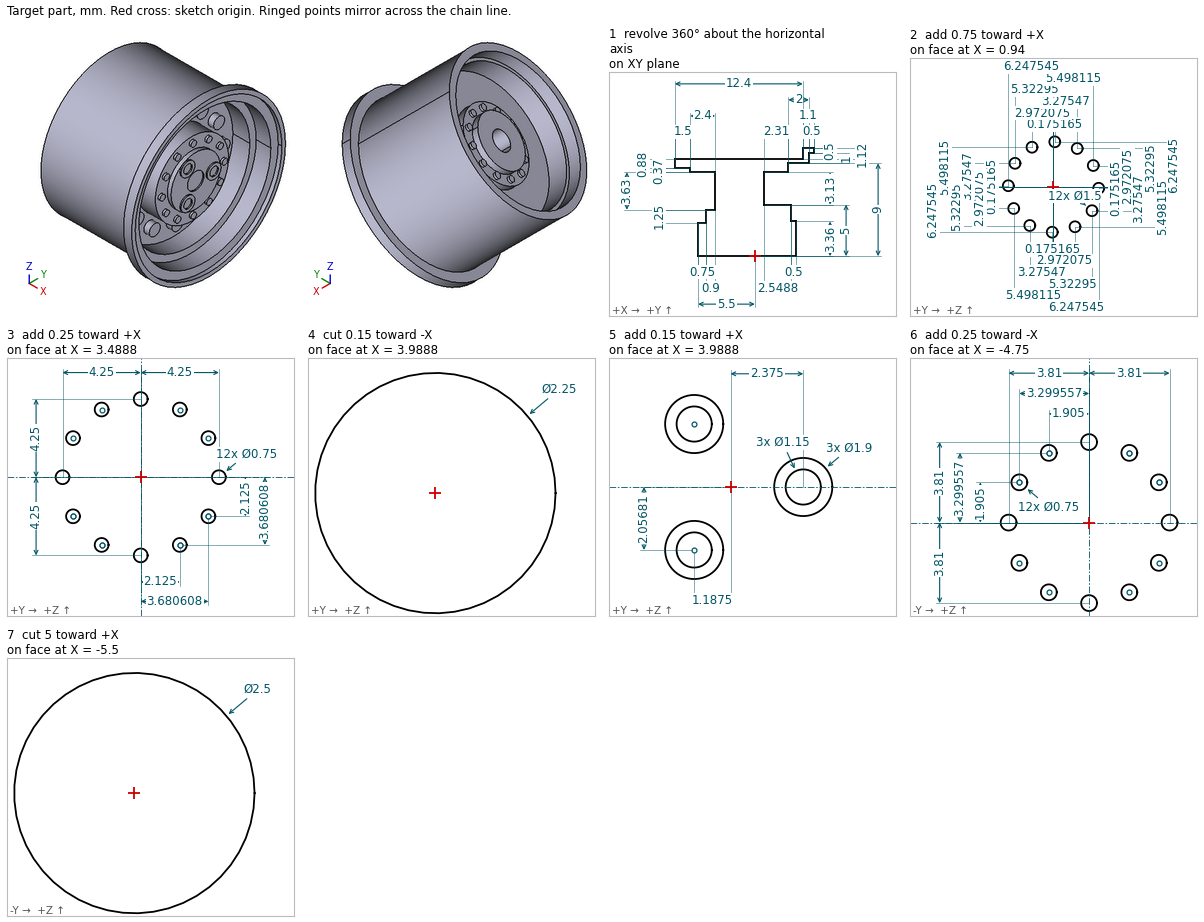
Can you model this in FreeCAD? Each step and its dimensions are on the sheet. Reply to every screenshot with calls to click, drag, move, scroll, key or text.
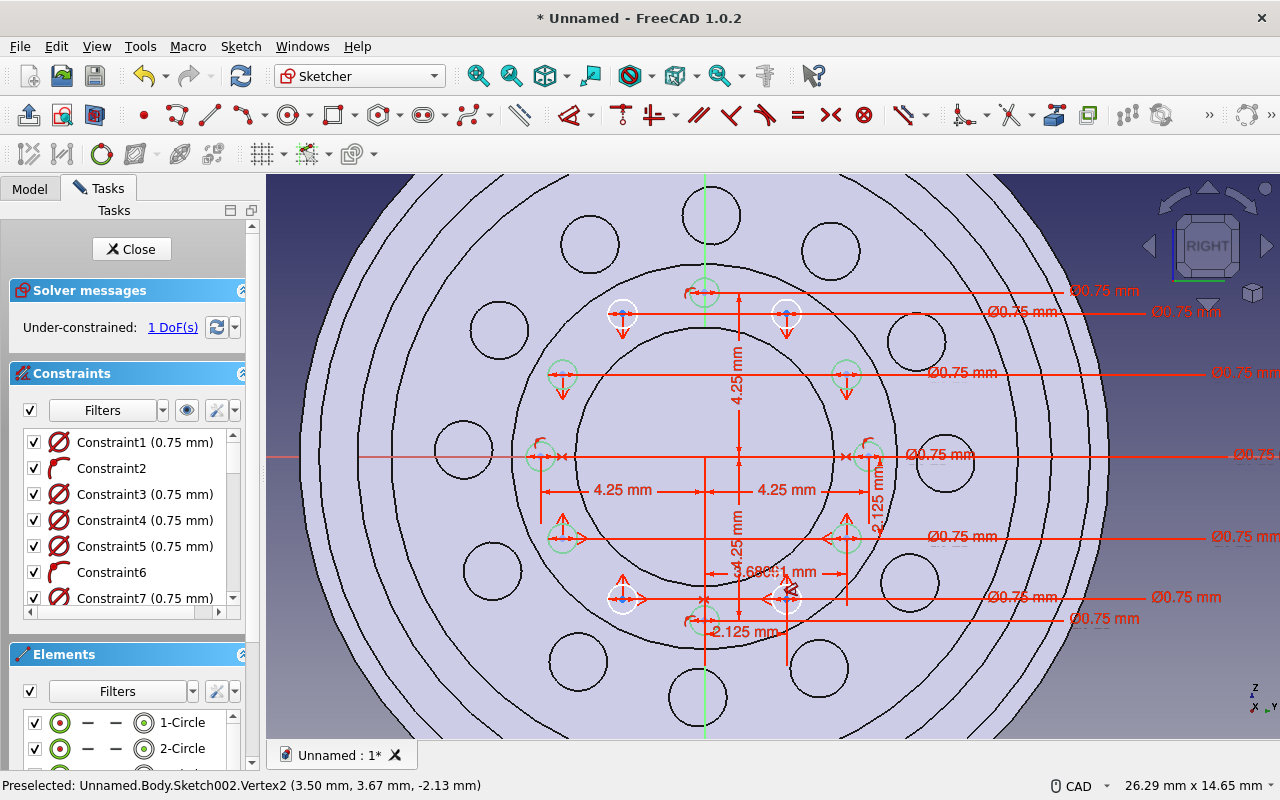
click(787, 599)
click(821, 528)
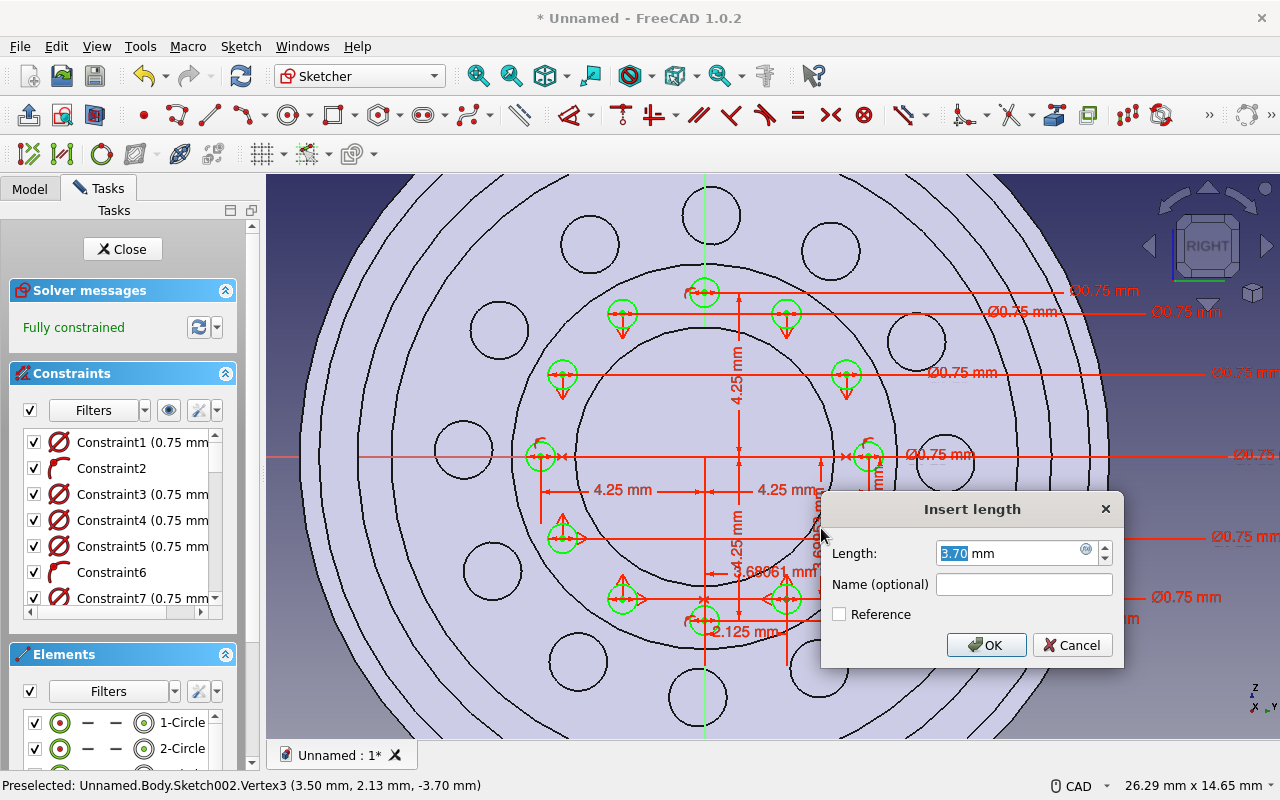
text(3.680608)
key(Return)
key(Escape)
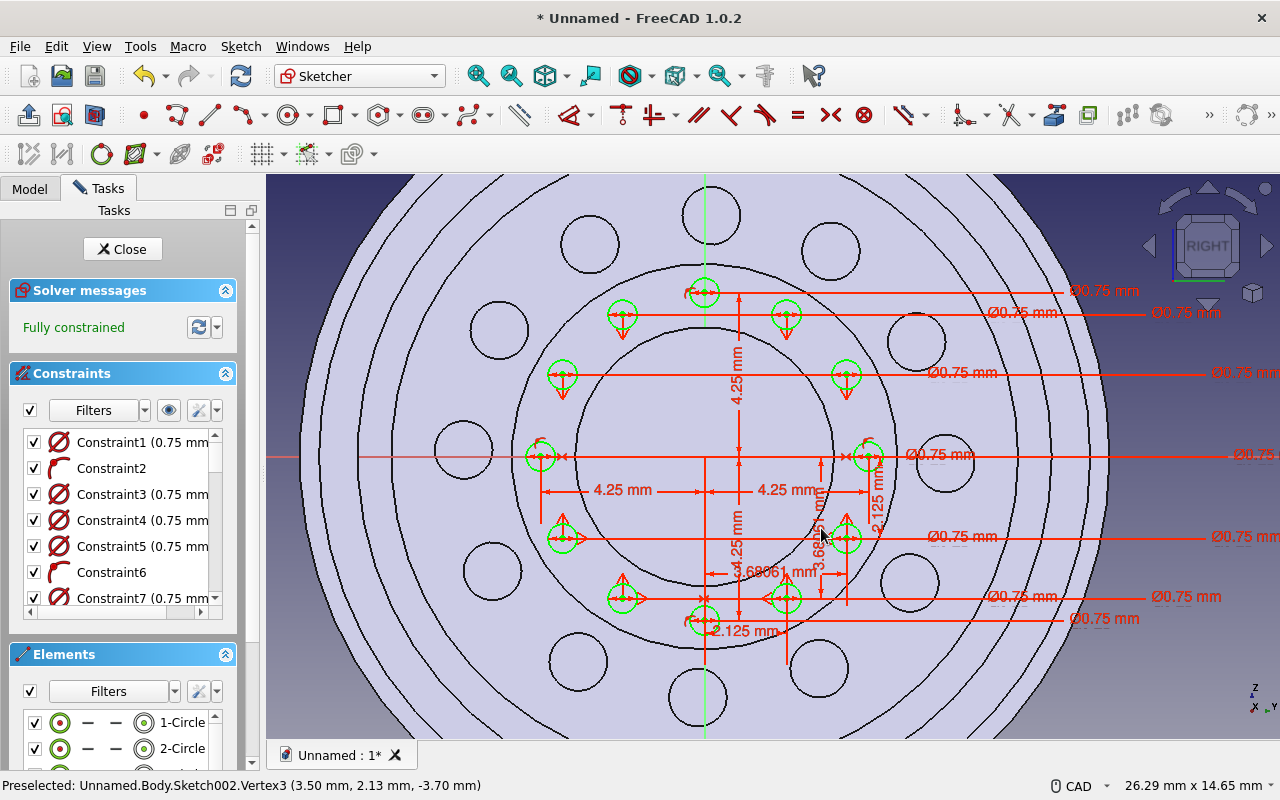
click(123, 249)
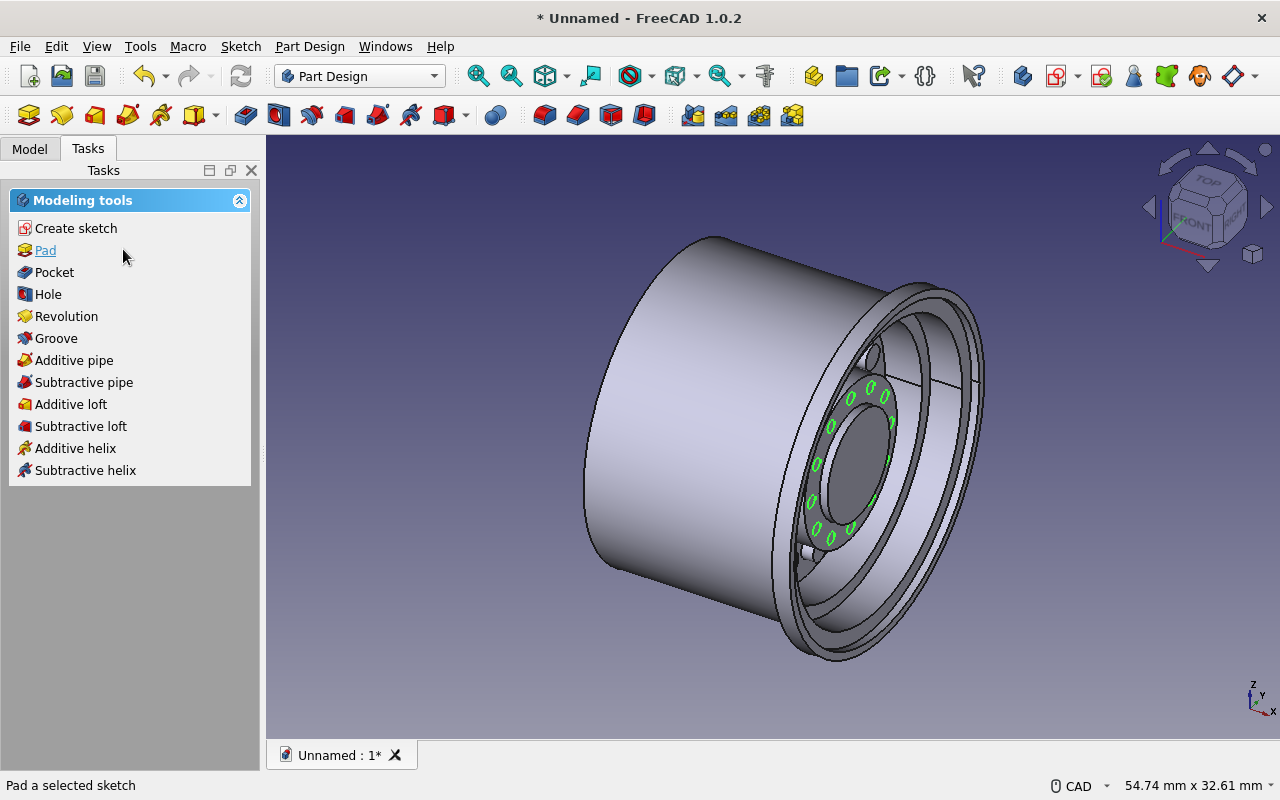
click(29, 116)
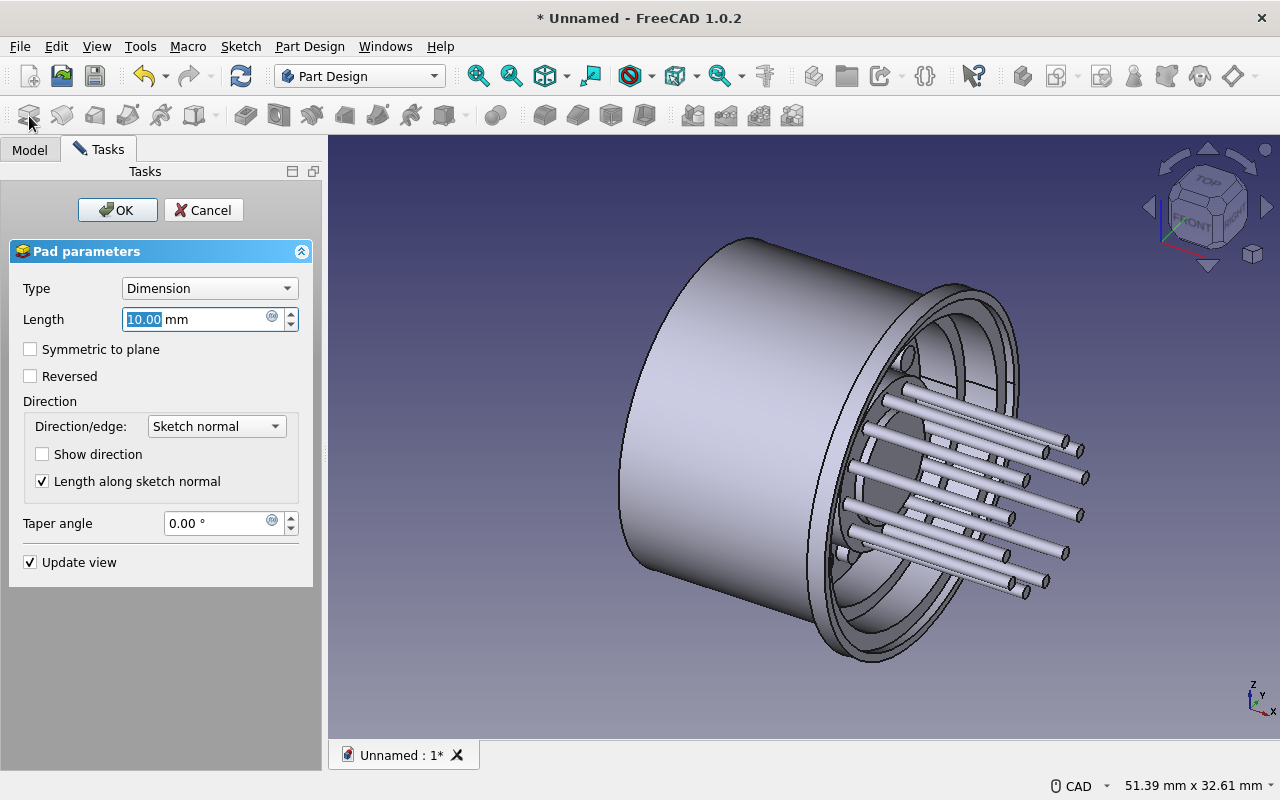
text(0.25)
key(Tab)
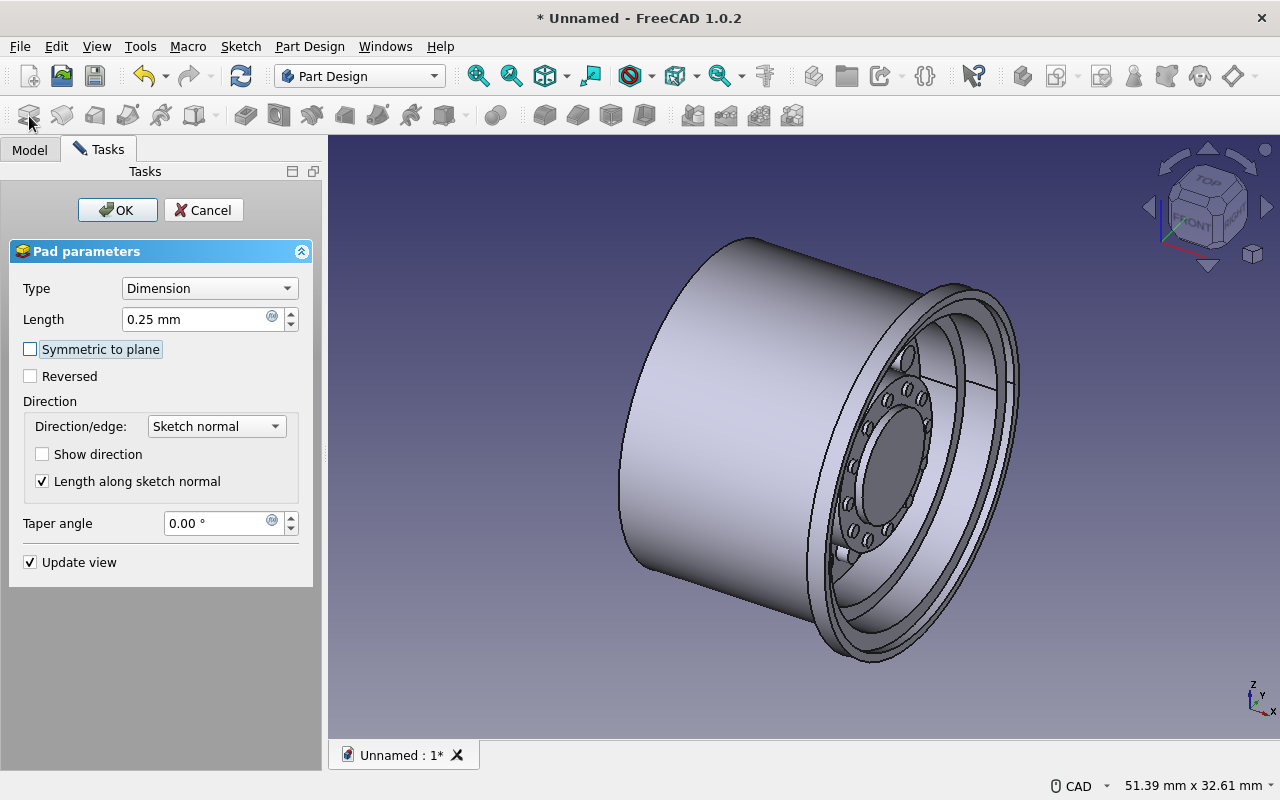
click(118, 210)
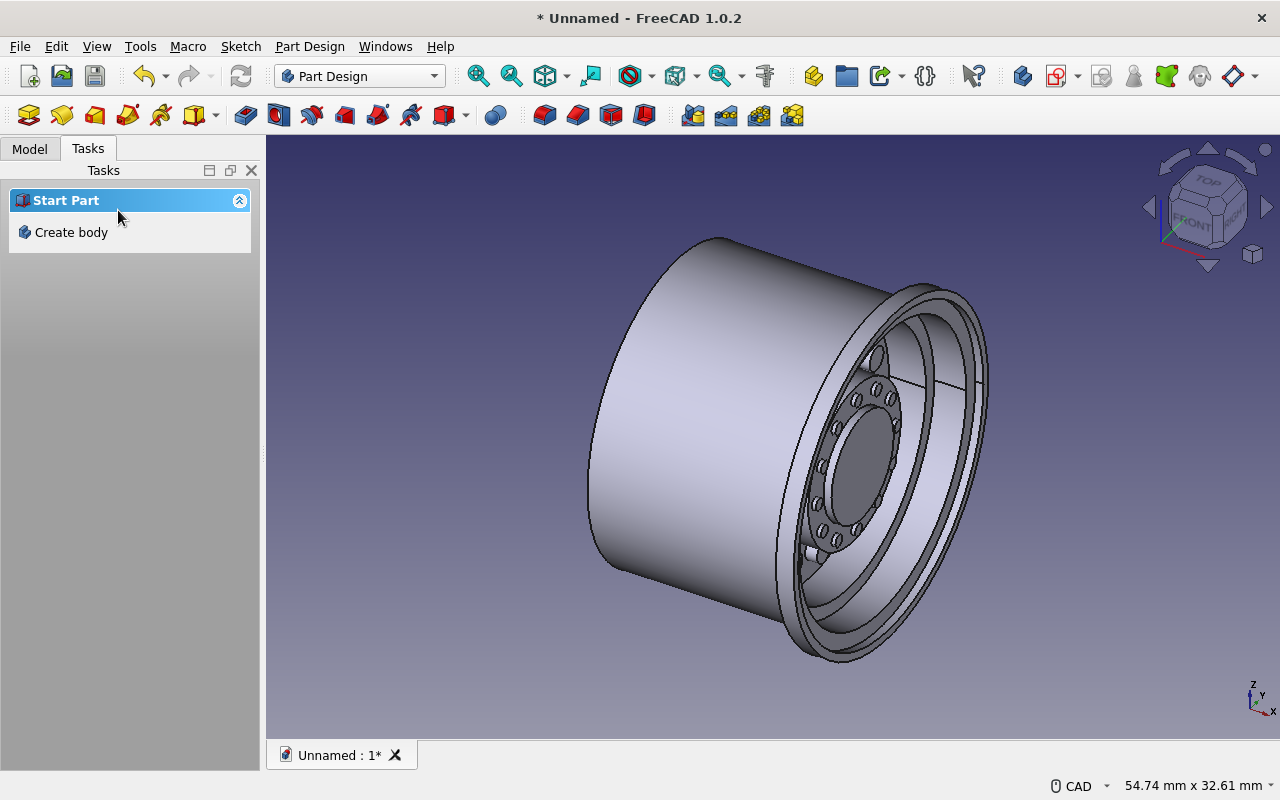
click(863, 466)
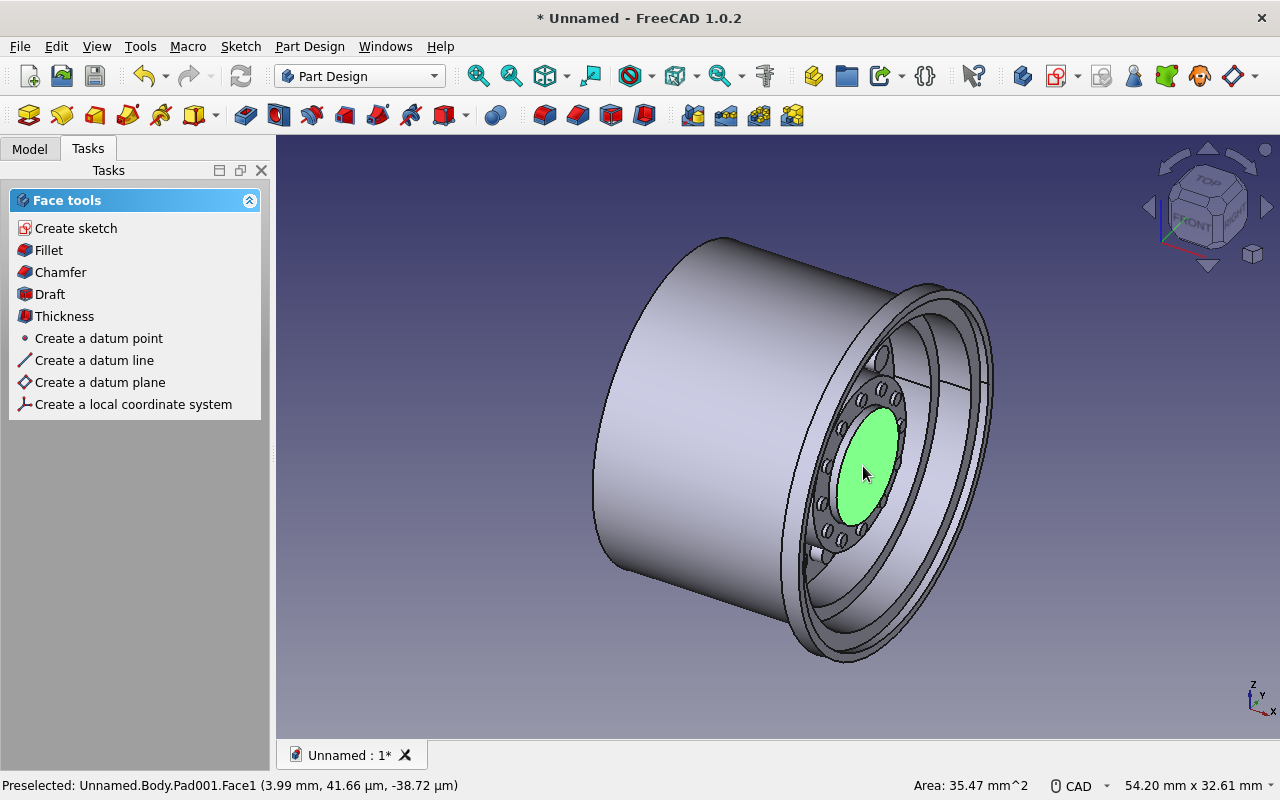
click(1056, 76)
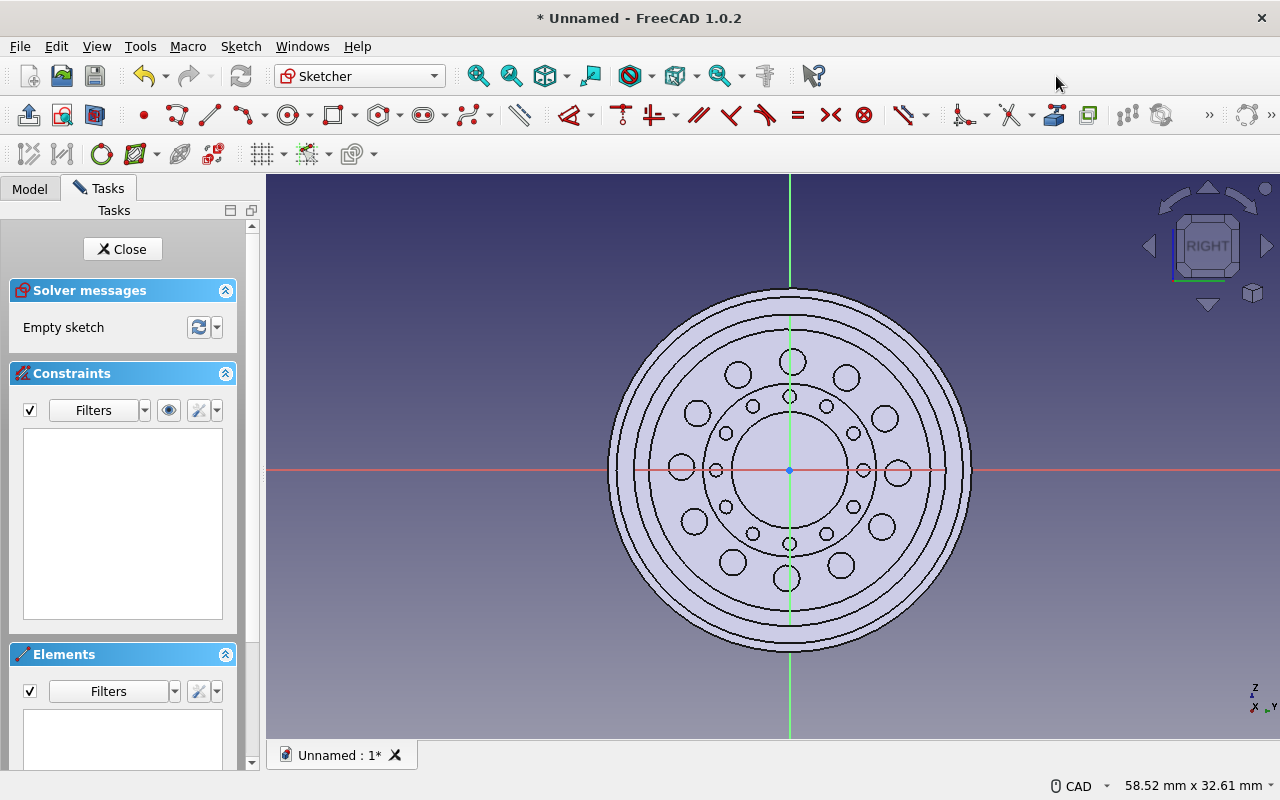
scroll(800, 472, up, 11)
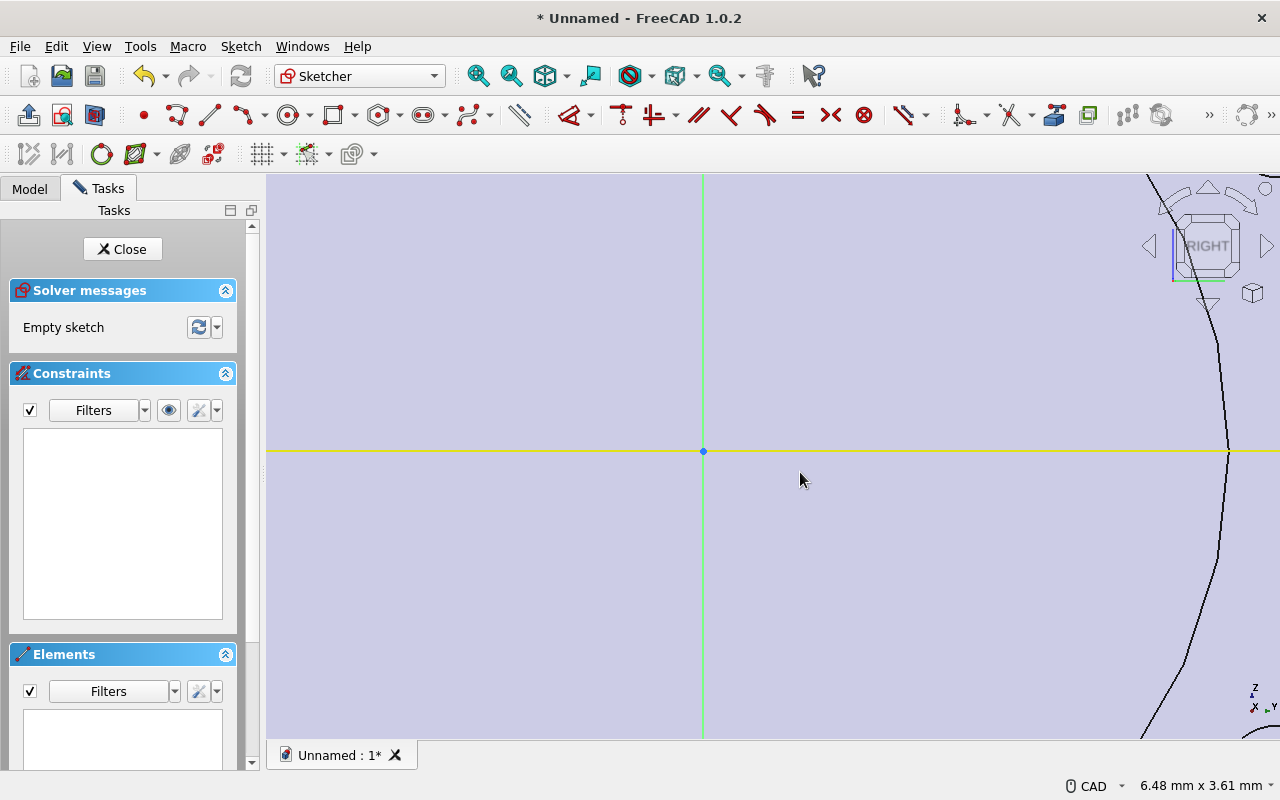
click(288, 116)